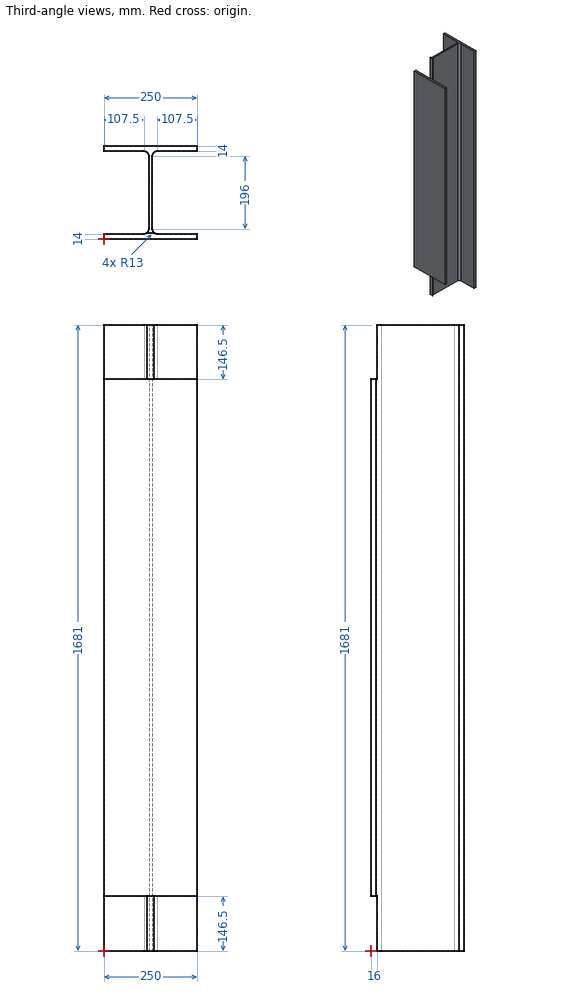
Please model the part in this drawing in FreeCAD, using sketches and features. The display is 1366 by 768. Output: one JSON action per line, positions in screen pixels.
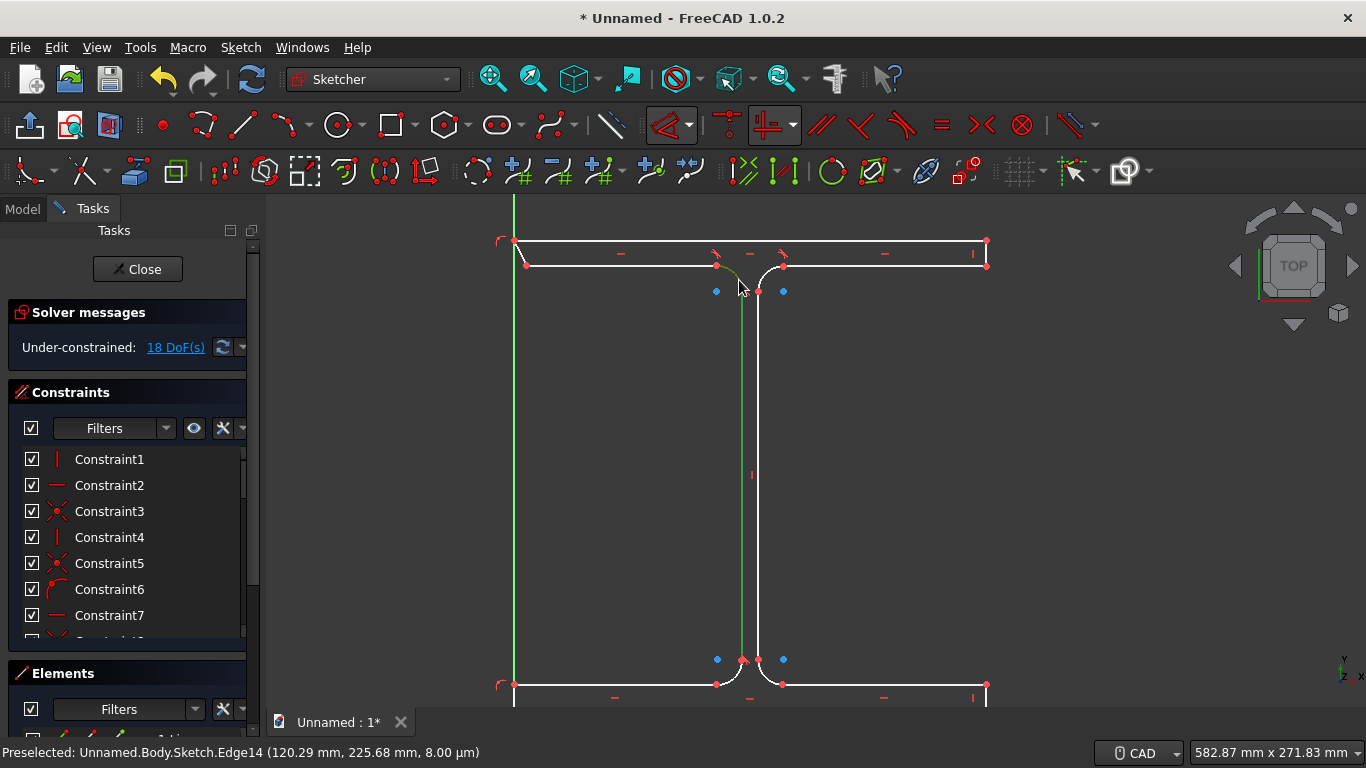
{"action": "left_click", "coordinate": [902, 126]}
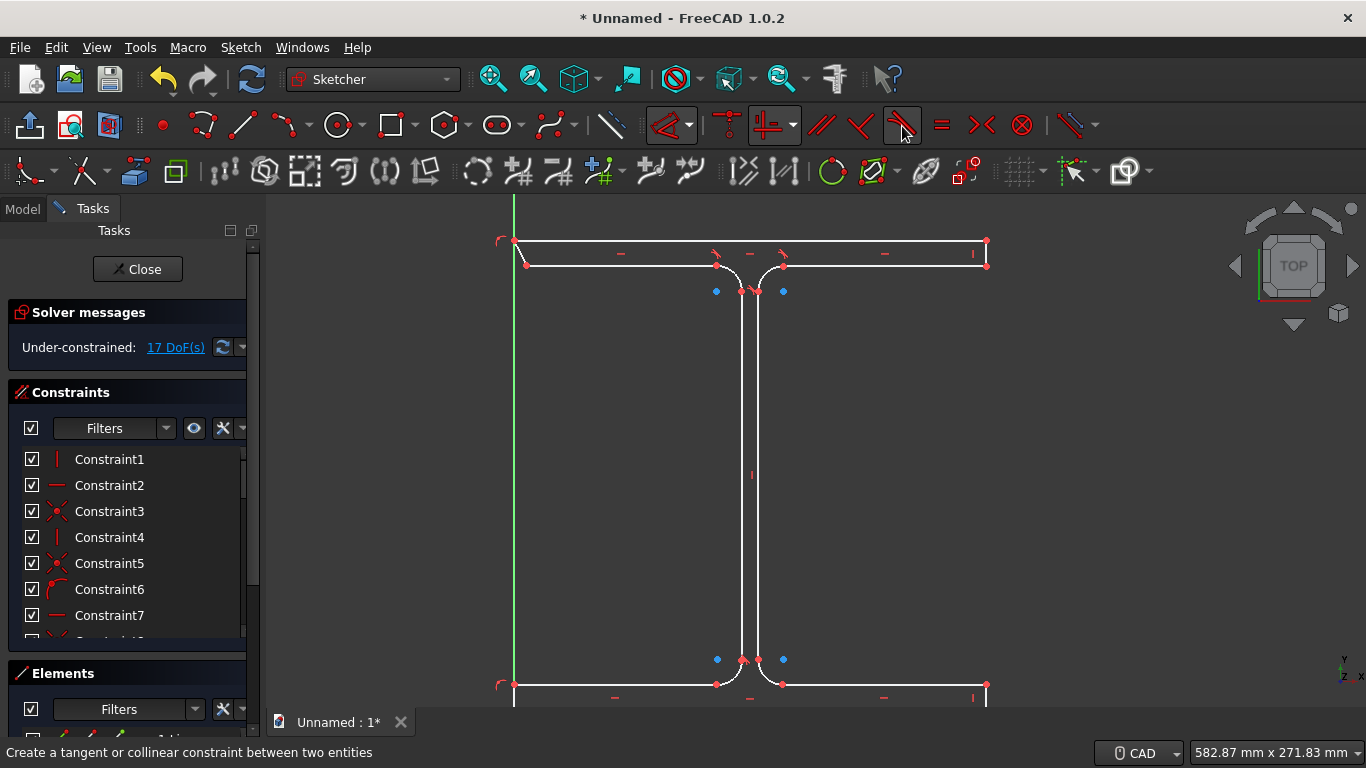
{"action": "left_click", "coordinate": [742, 402]}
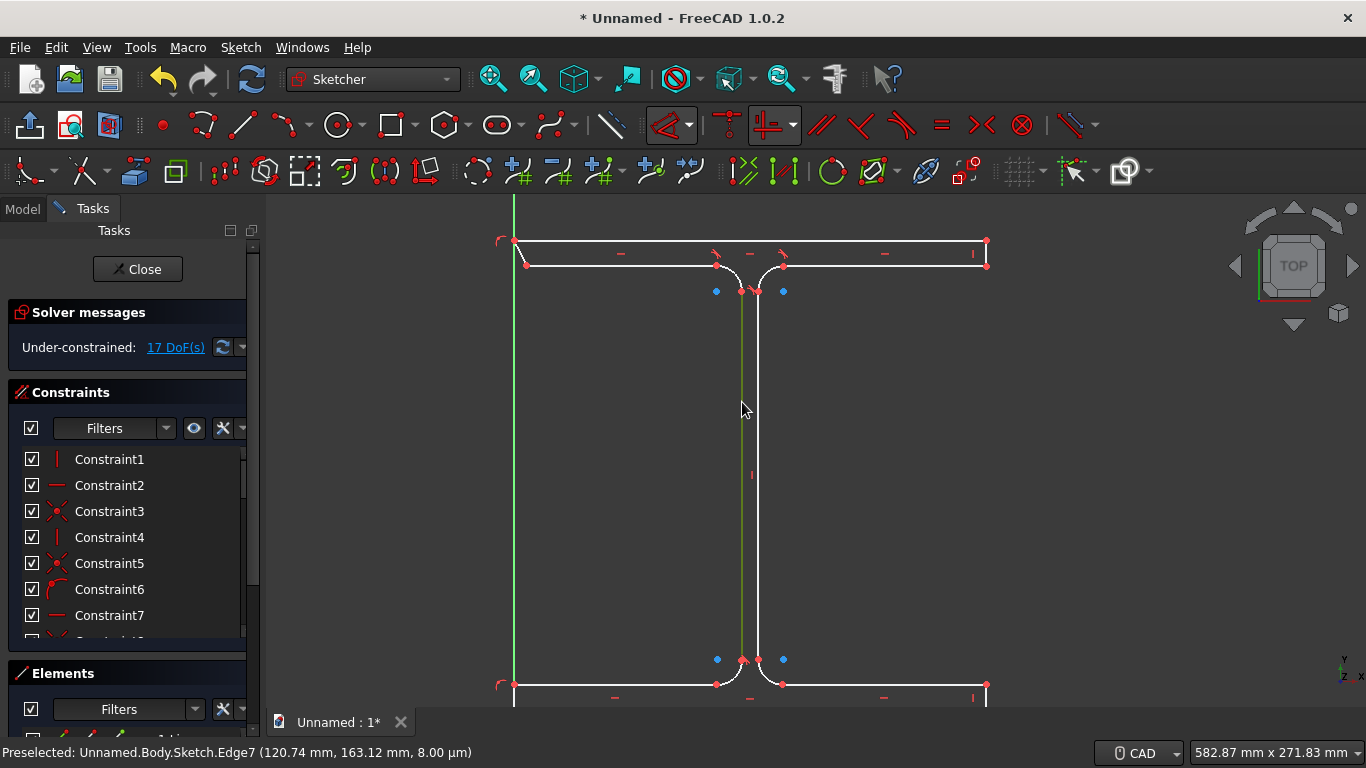
{"action": "left_click", "coordinate": [739, 672]}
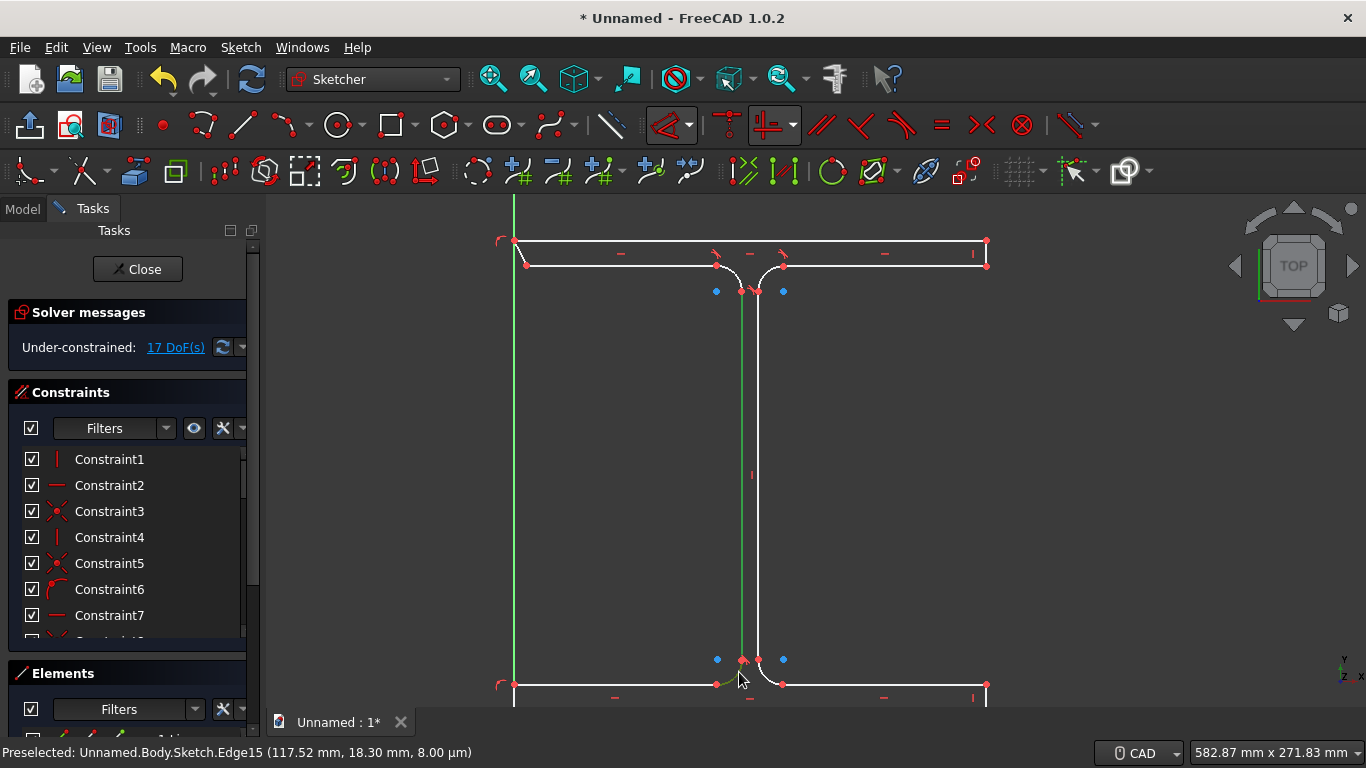
{"action": "left_click", "coordinate": [902, 126]}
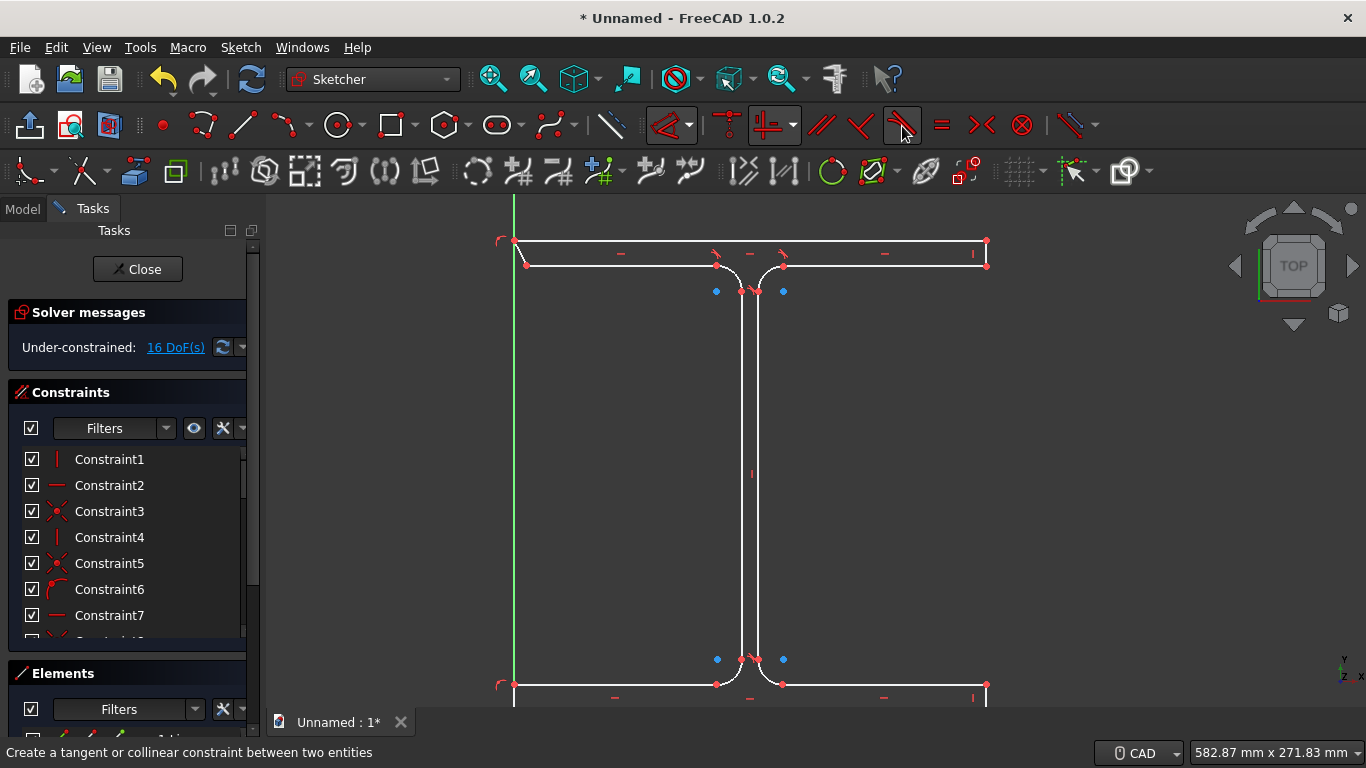
{"action": "scroll", "coordinate": [742, 401], "scroll_direction": "down", "scroll_amount": 2}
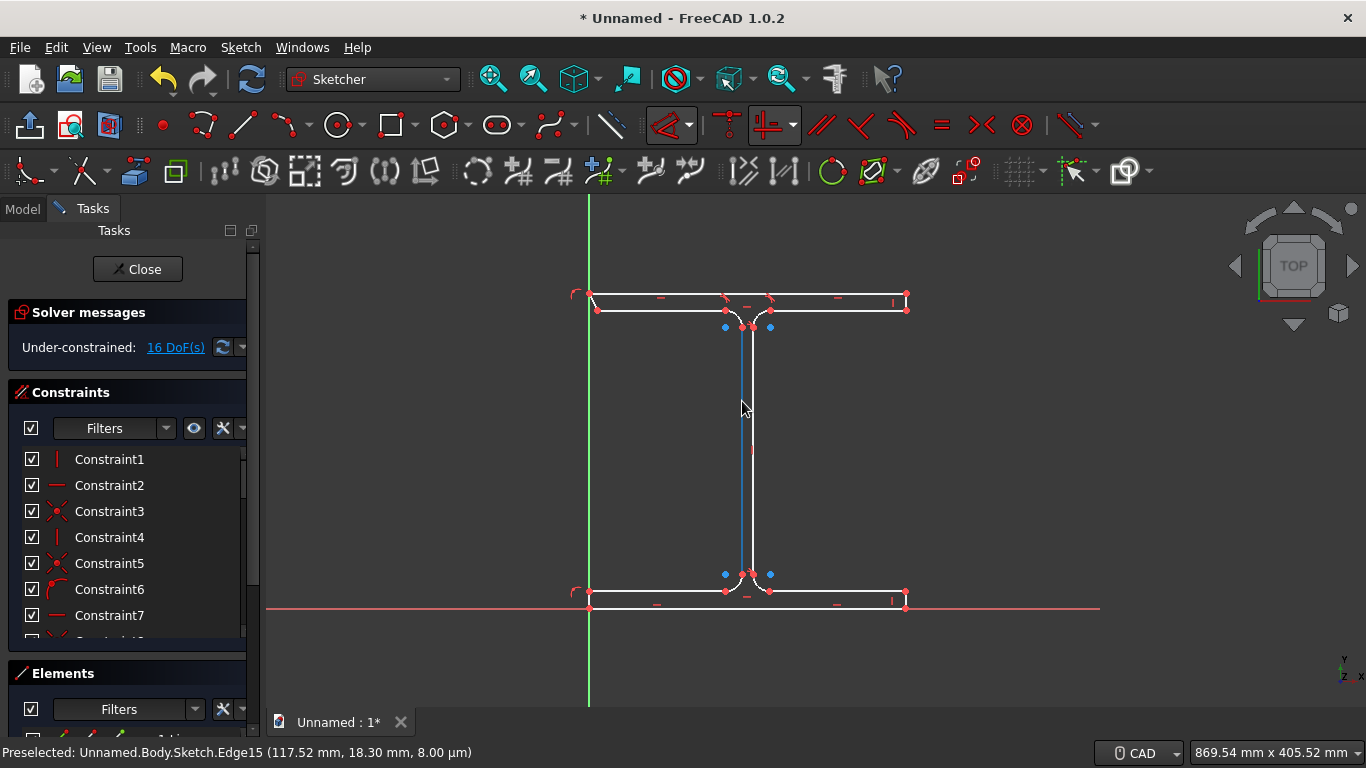
{"action": "left_click", "coordinate": [685, 591]}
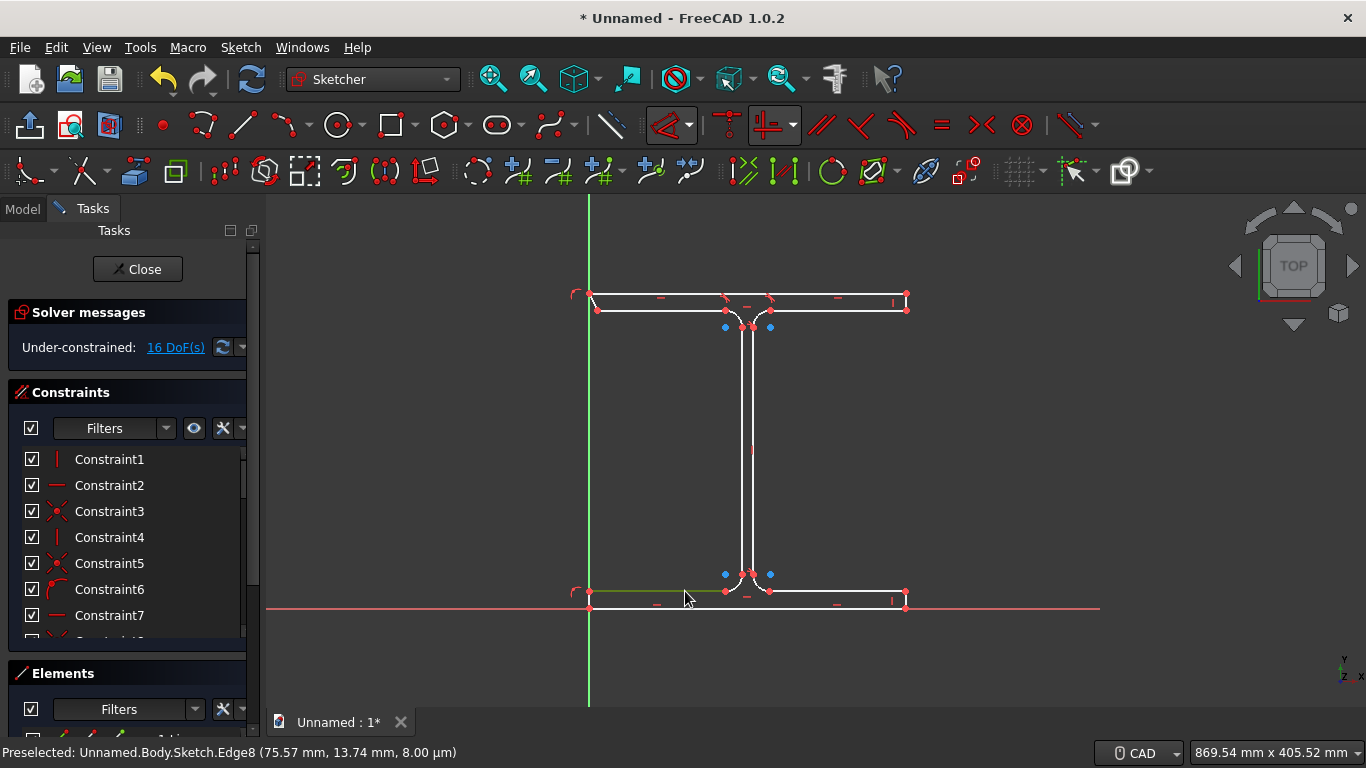
{"action": "left_click", "coordinate": [737, 587]}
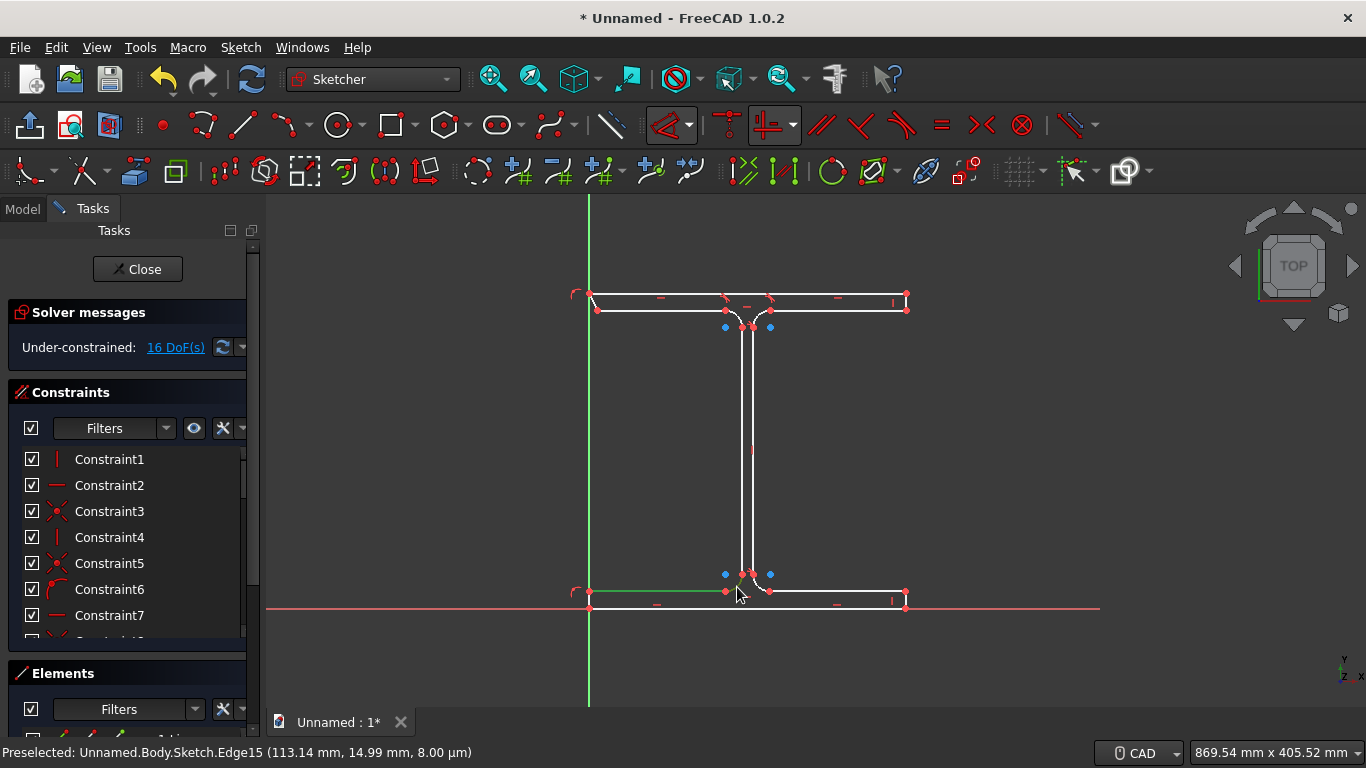
{"action": "left_click", "coordinate": [902, 126]}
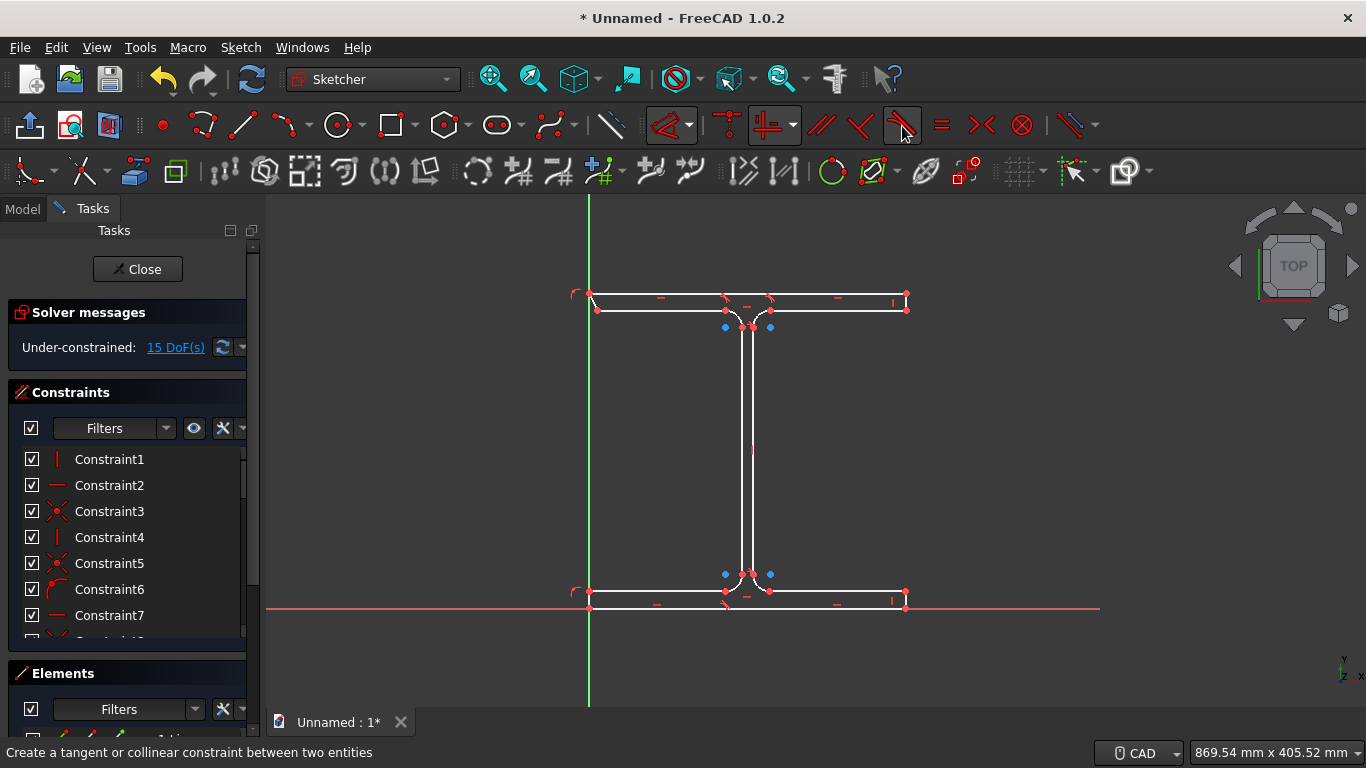
{"action": "left_click", "coordinate": [865, 591]}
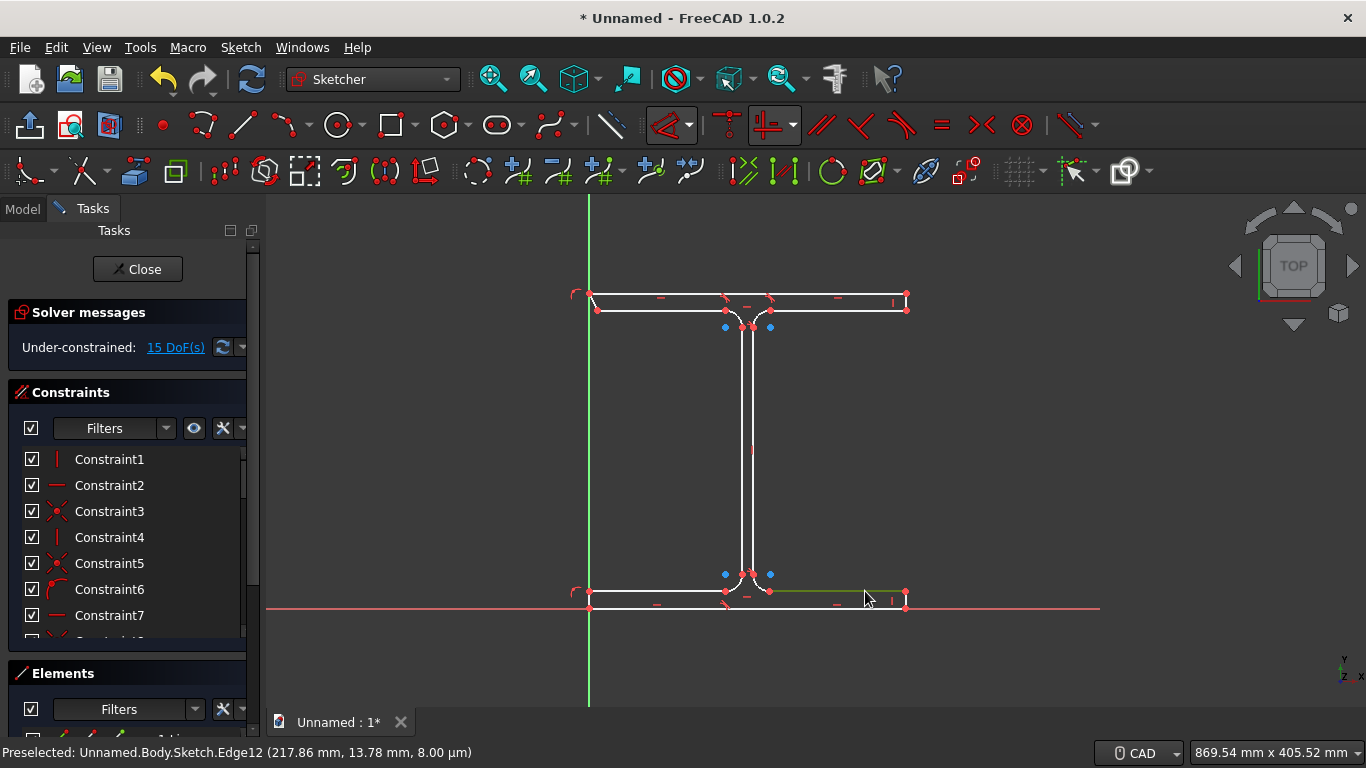
{"action": "left_click", "coordinate": [758, 586]}